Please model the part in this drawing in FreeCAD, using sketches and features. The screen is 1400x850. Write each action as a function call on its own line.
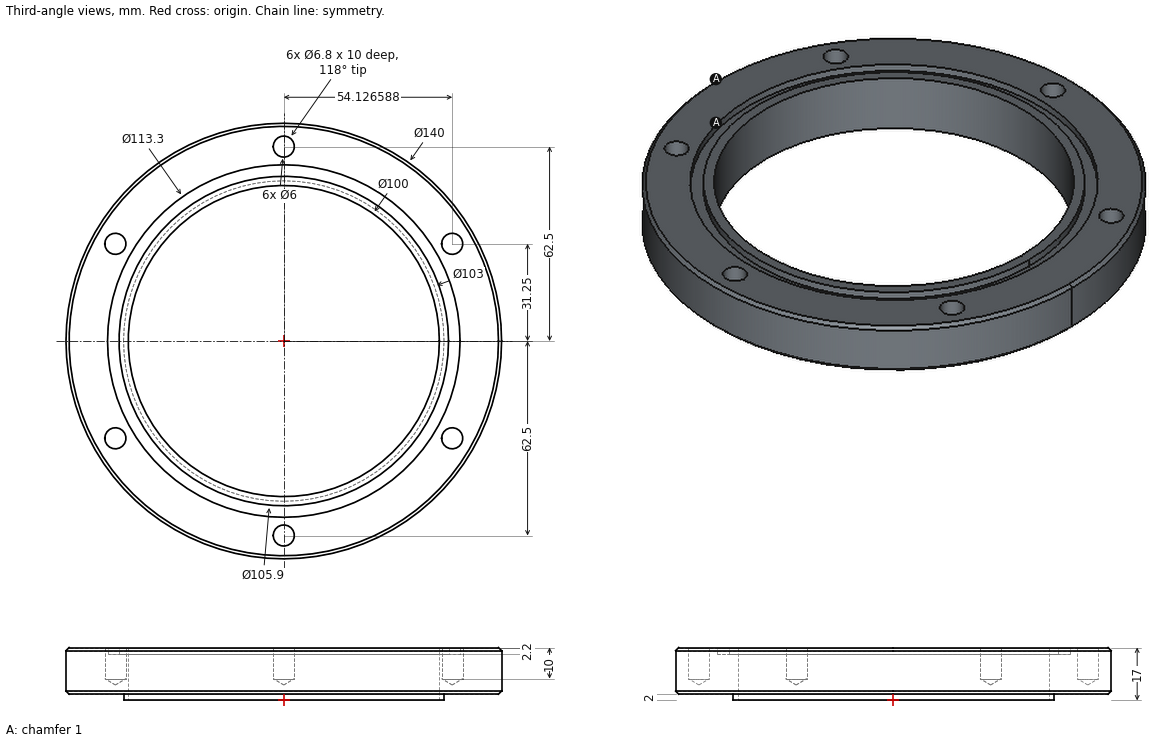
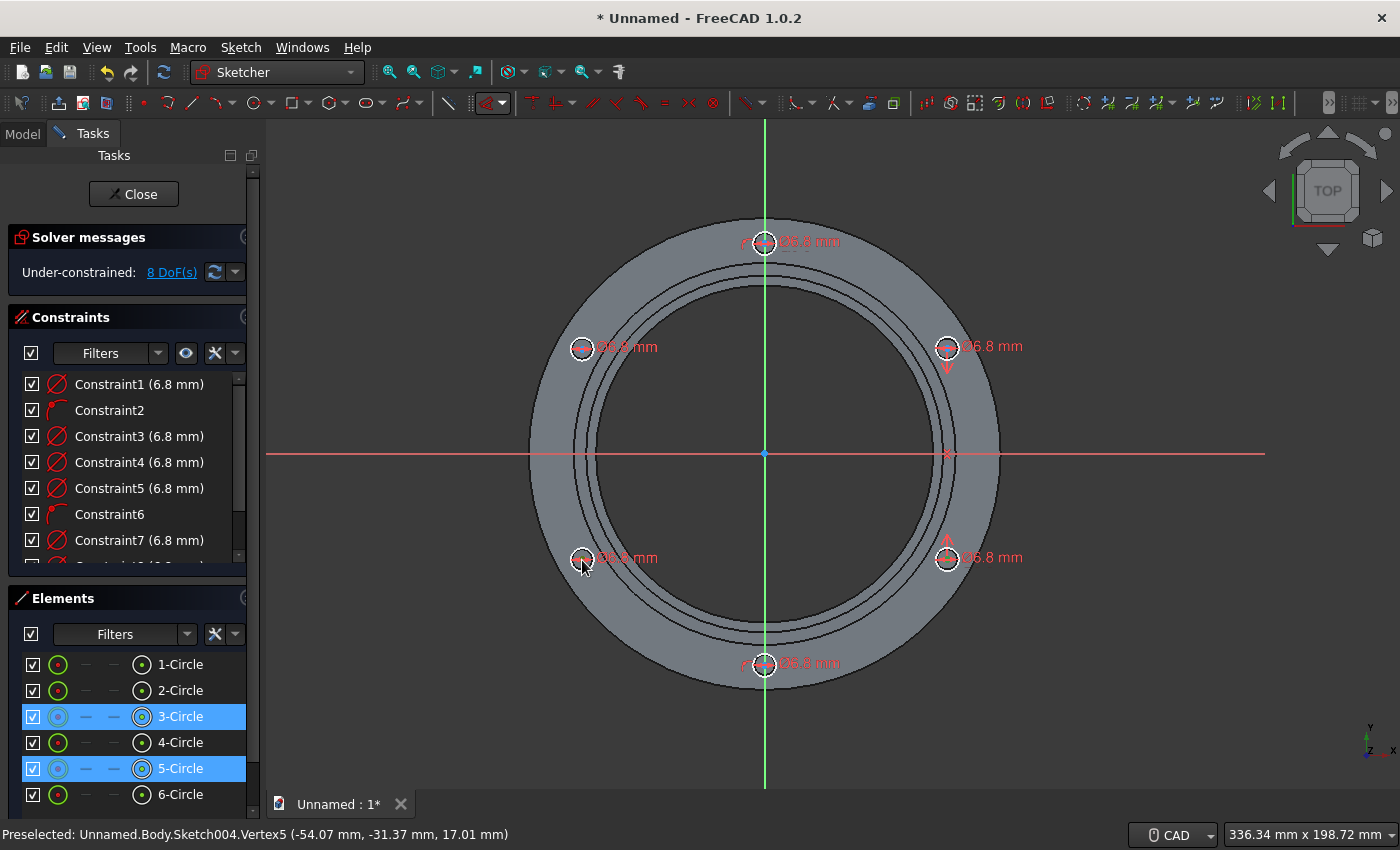
click(765, 717)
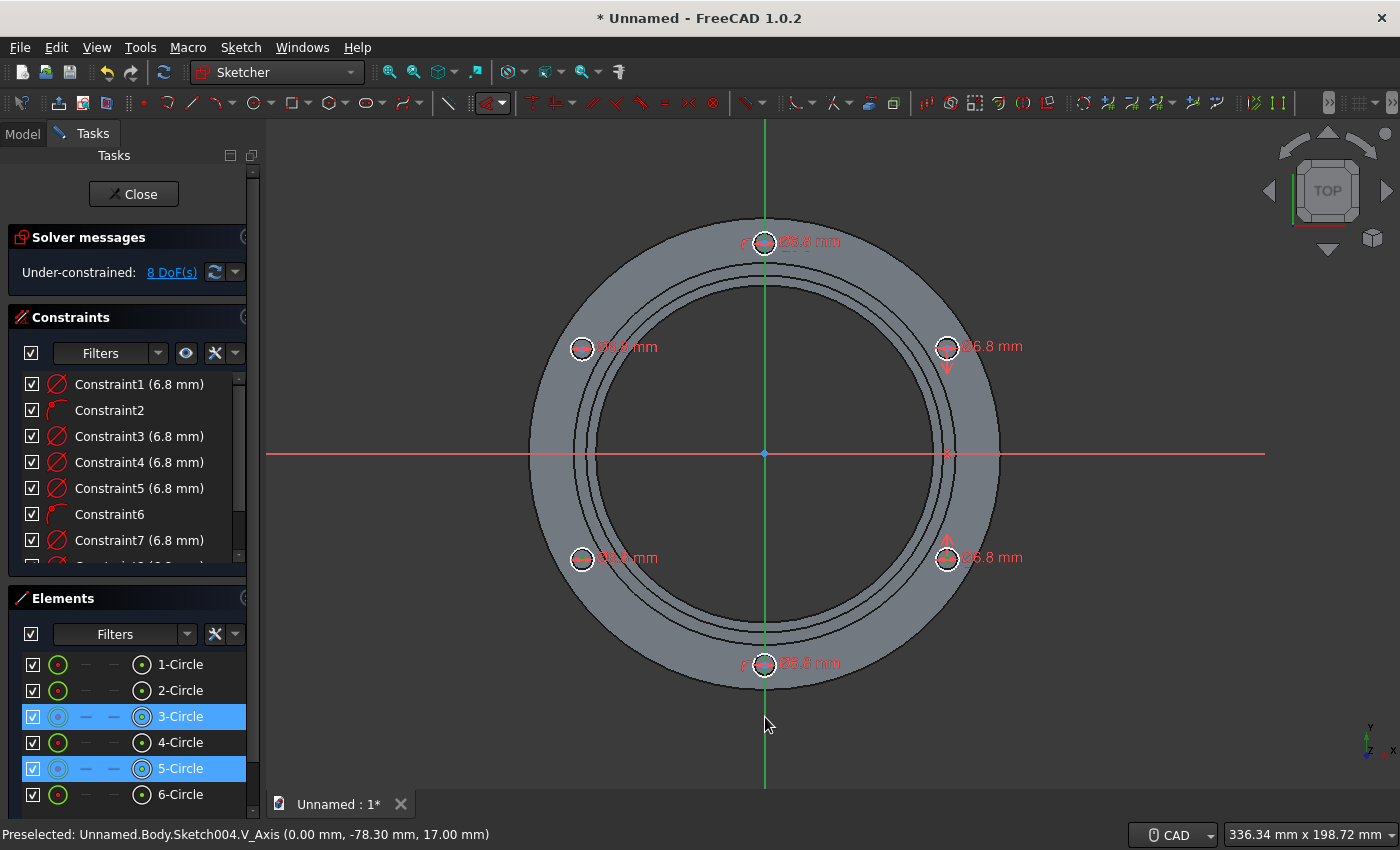
click(690, 104)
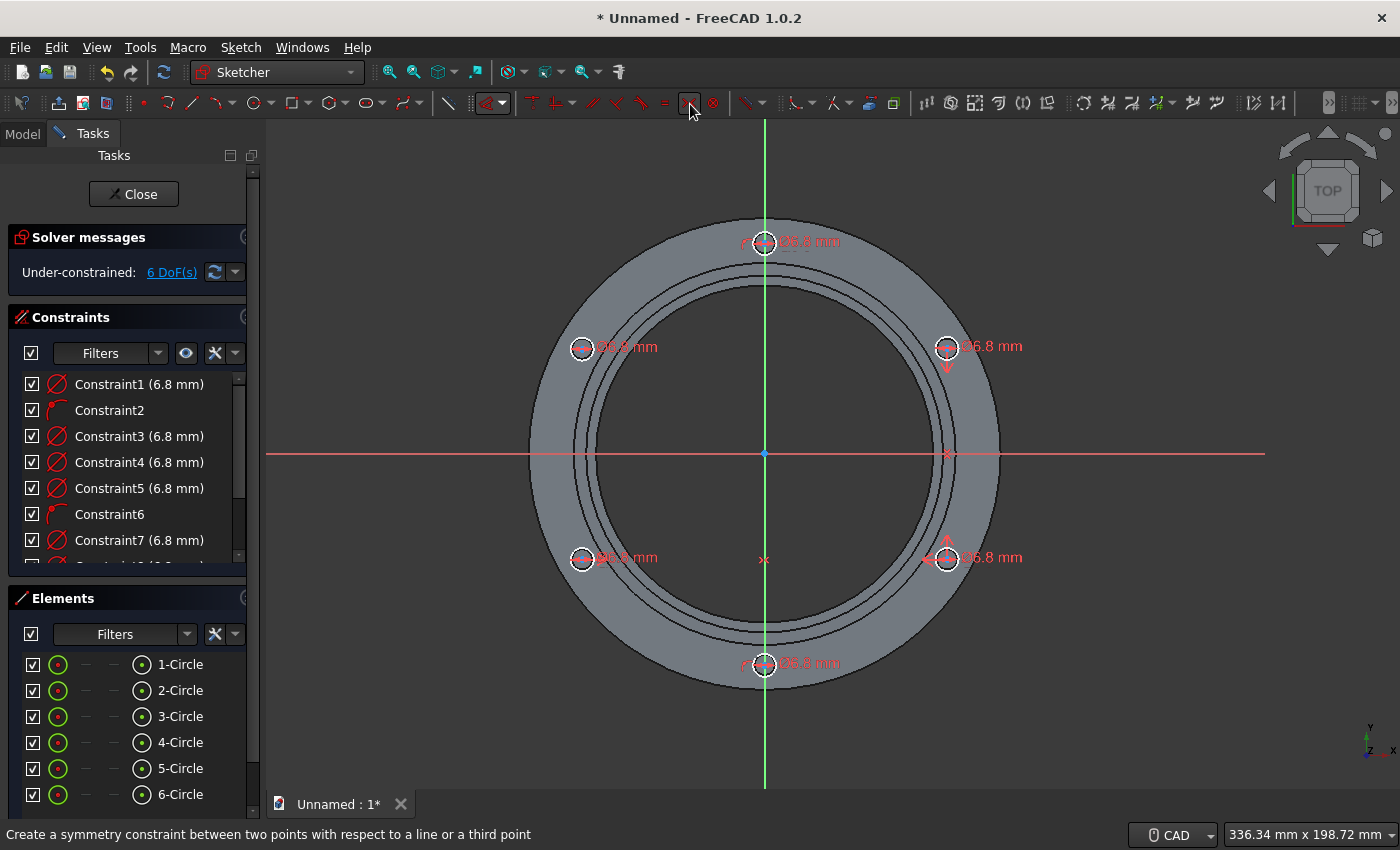
click(947, 348)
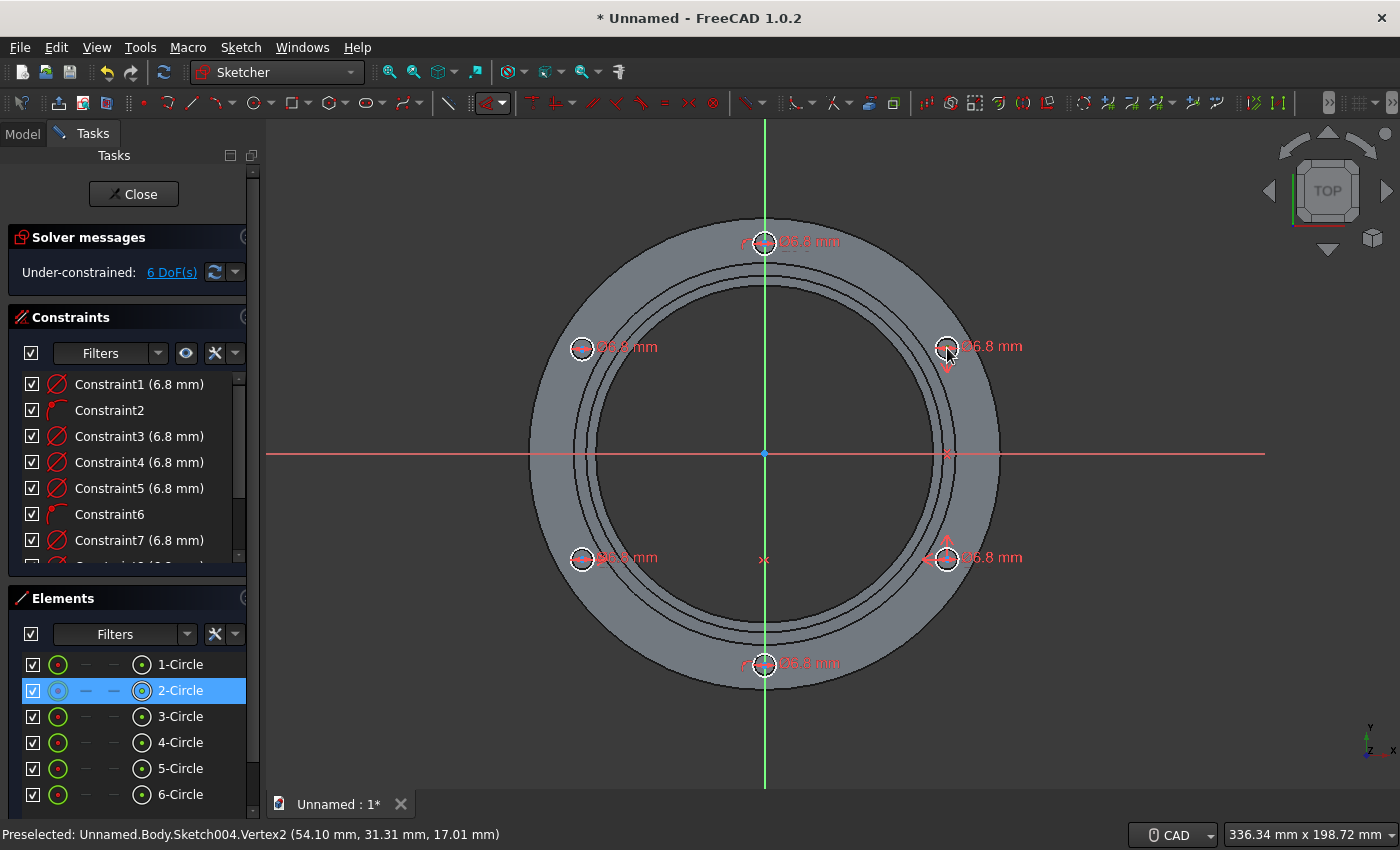
click(582, 349)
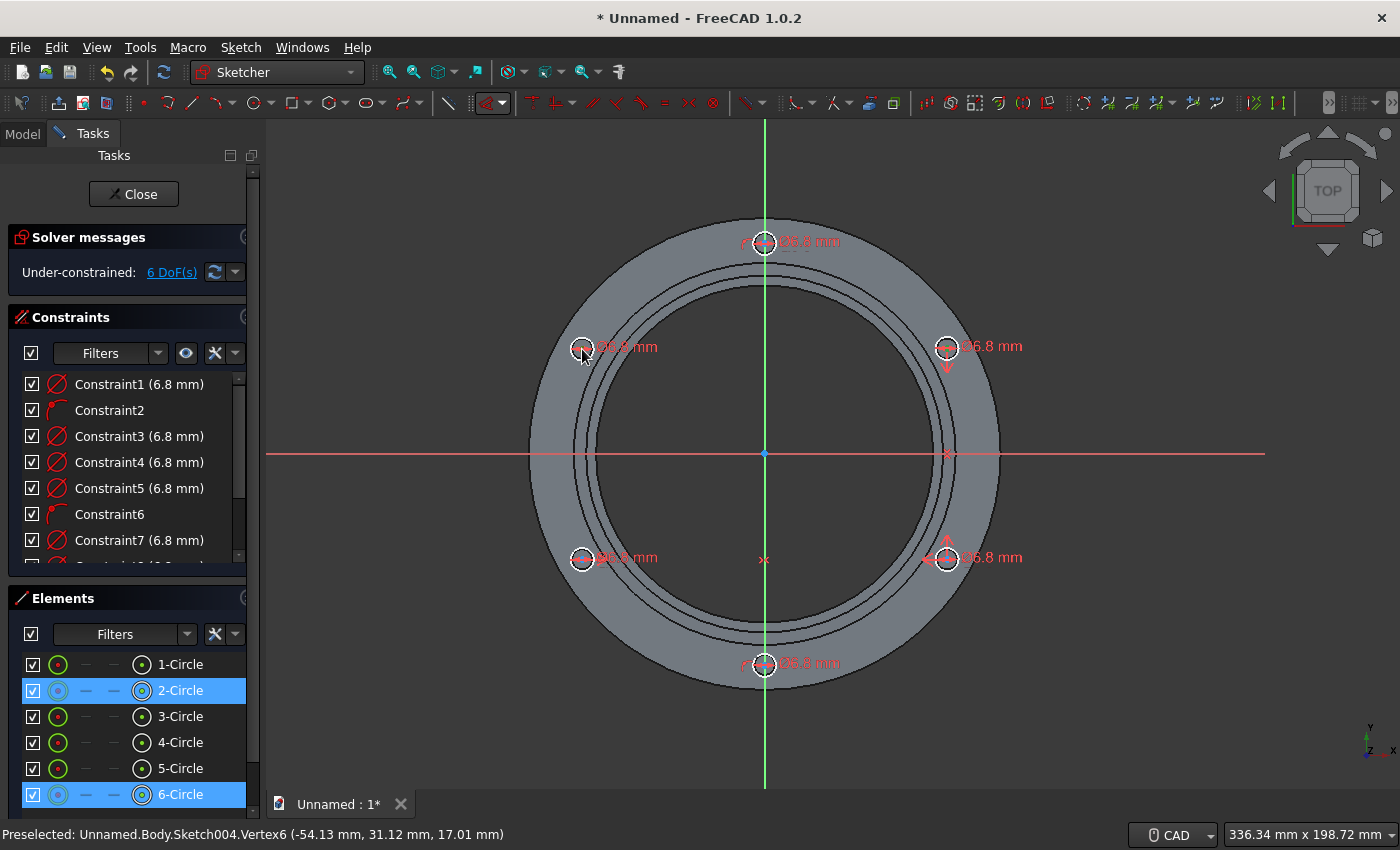
click(765, 717)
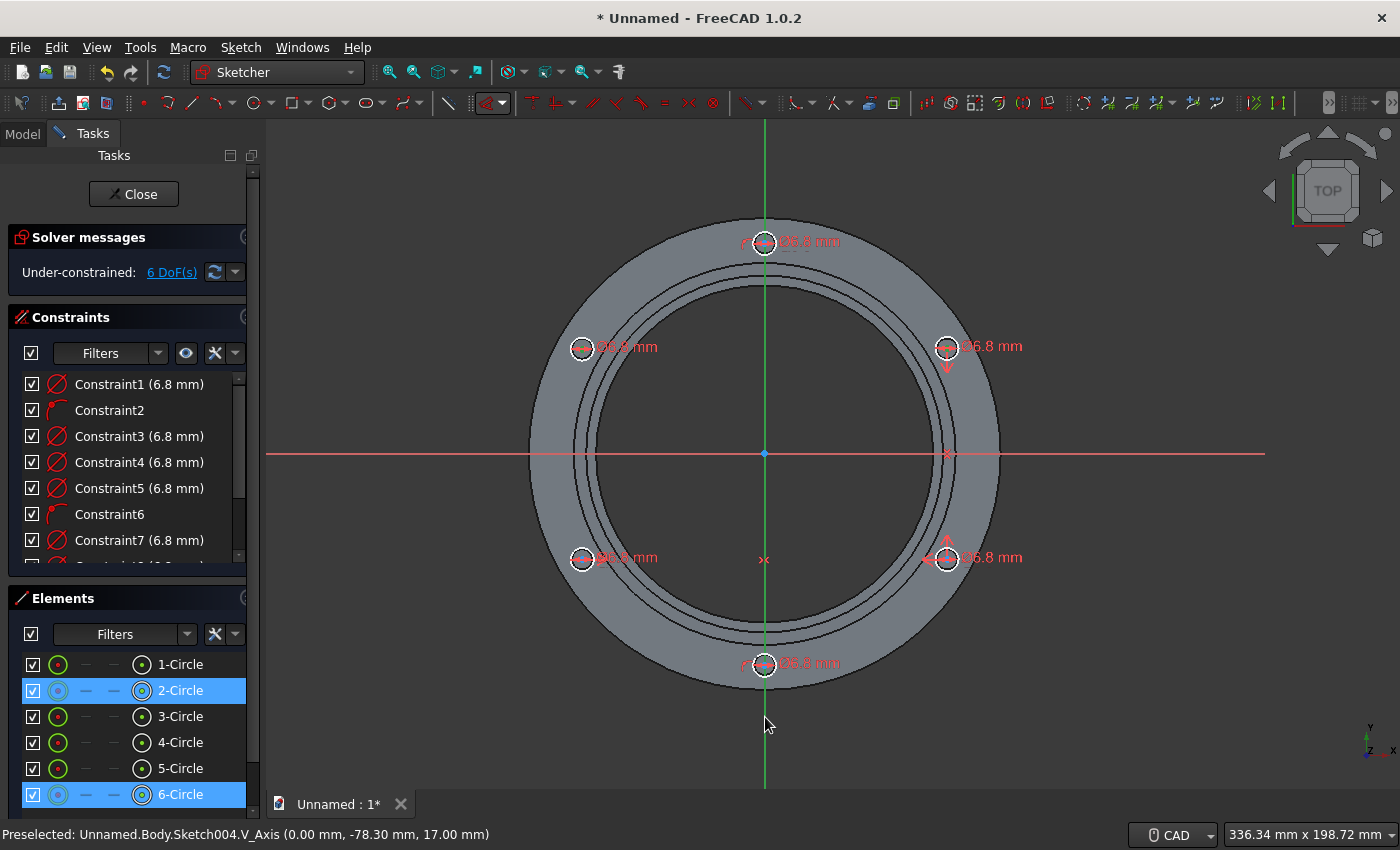
click(690, 104)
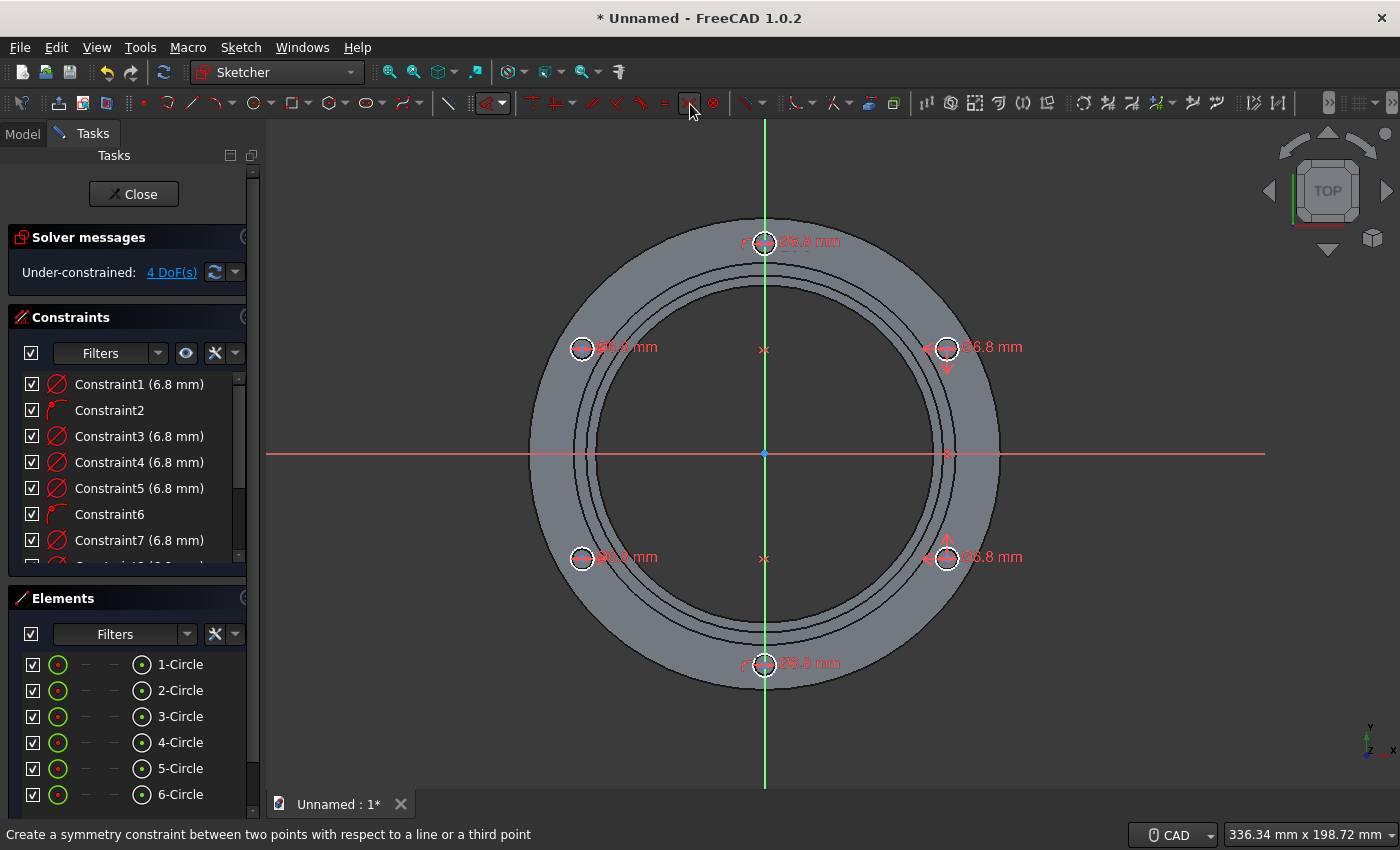
click(765, 244)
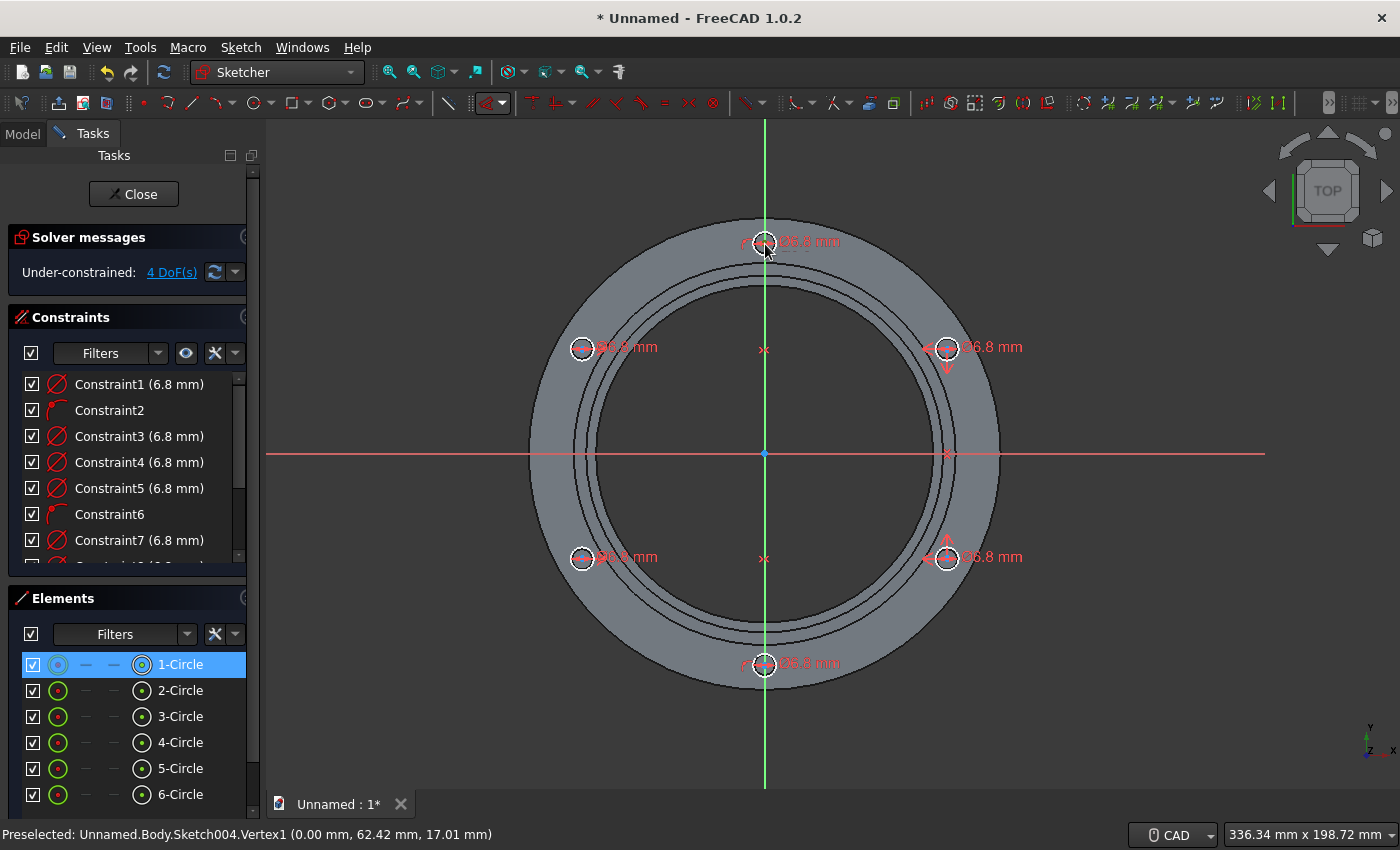
click(504, 104)